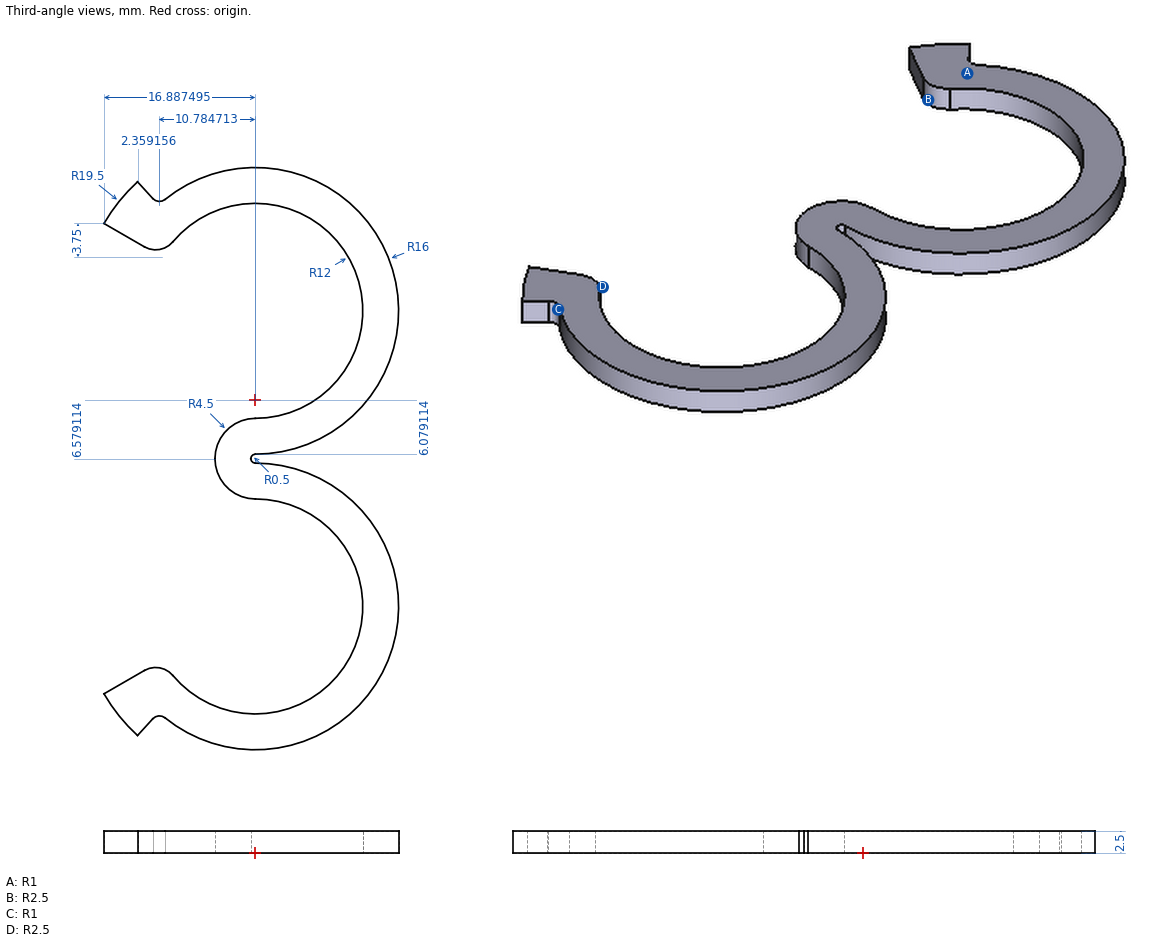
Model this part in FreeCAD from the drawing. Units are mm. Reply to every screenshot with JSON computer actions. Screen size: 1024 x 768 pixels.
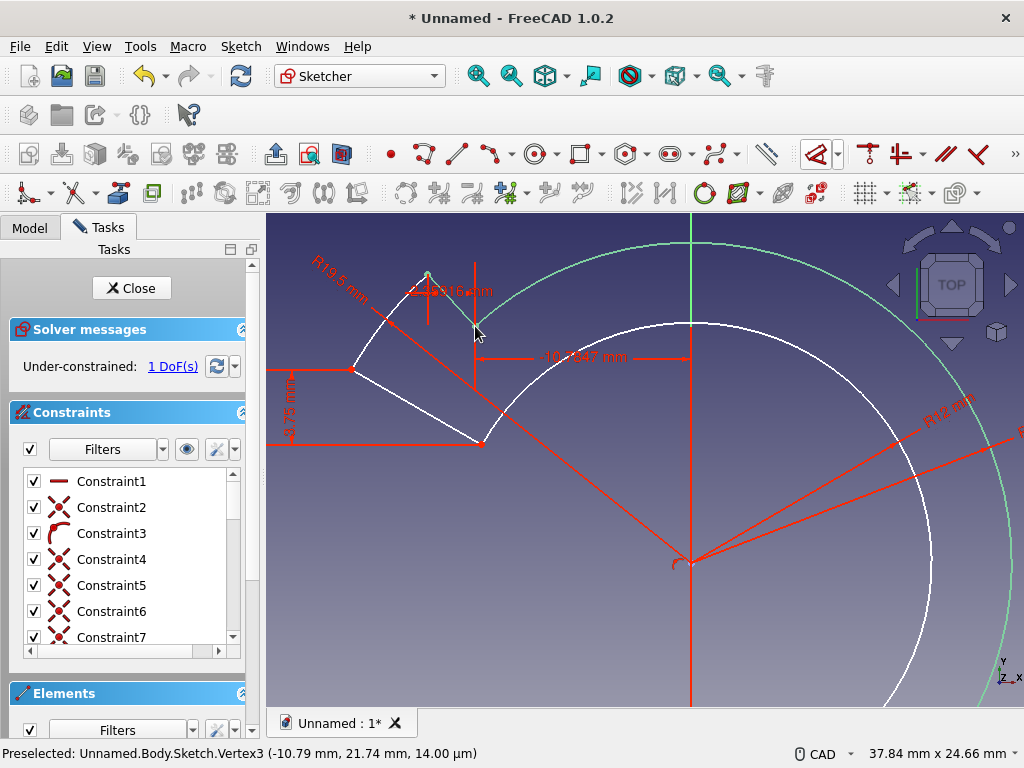
{"action": "left_click", "coordinate": [352, 370]}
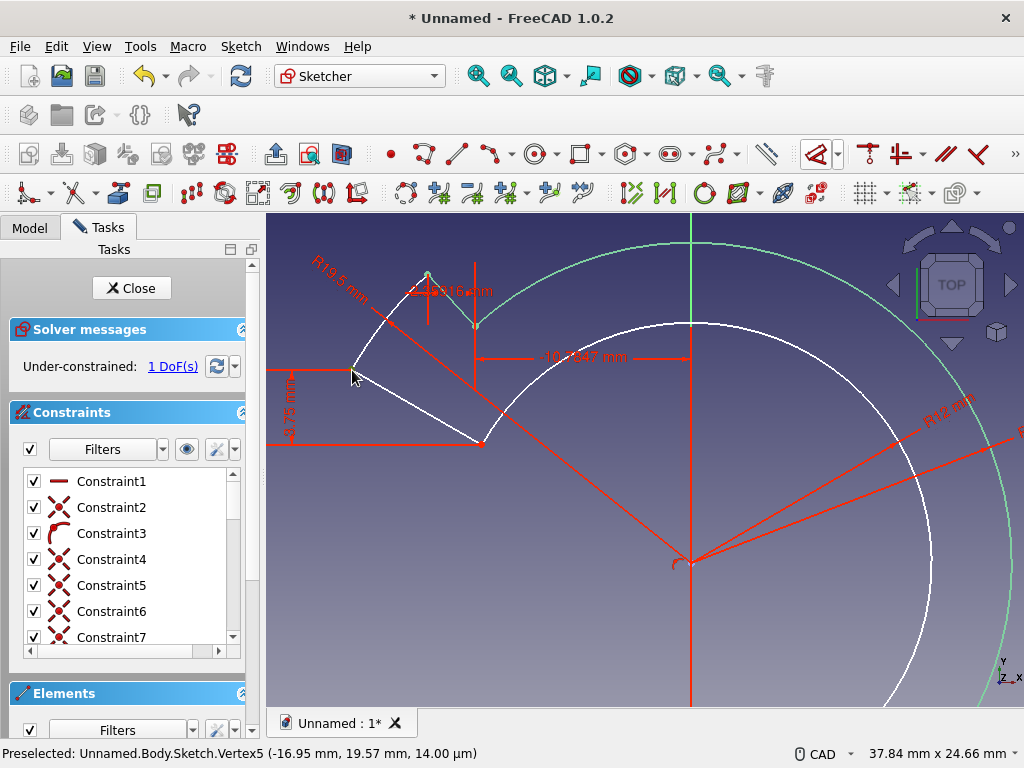
{"action": "left_click", "coordinate": [838, 154]}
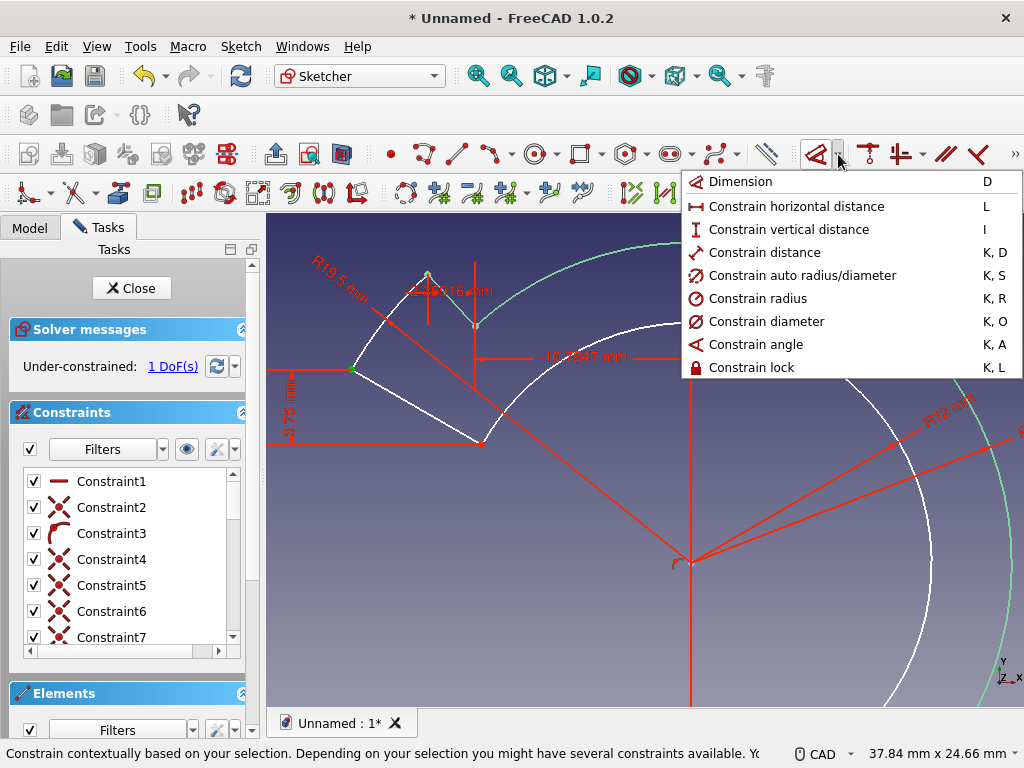
{"action": "left_click", "coordinate": [852, 206]}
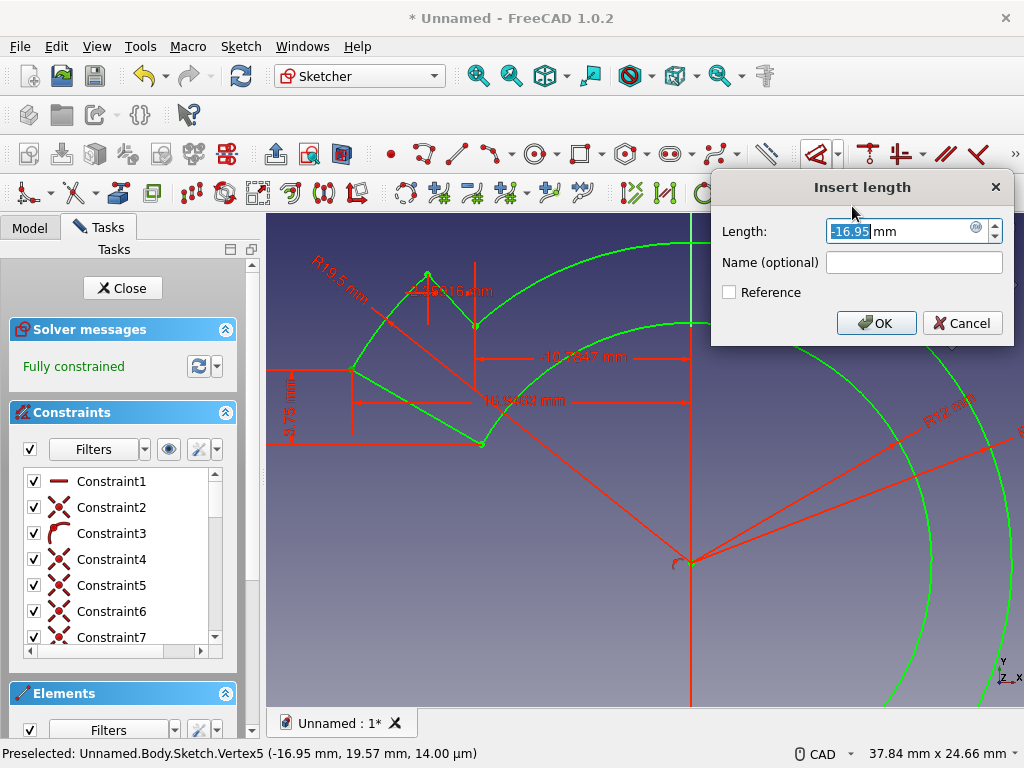
{"action": "type", "text": "-16.887495"}
{"action": "key", "text": "Return"}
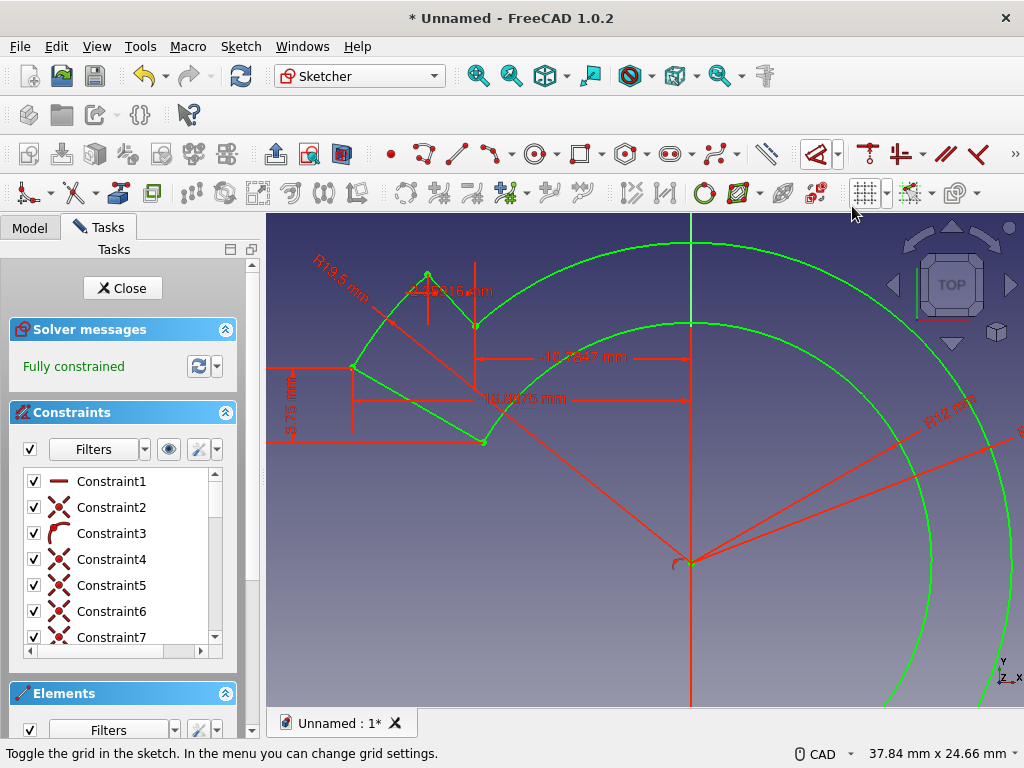
{"action": "left_click", "coordinate": [123, 288]}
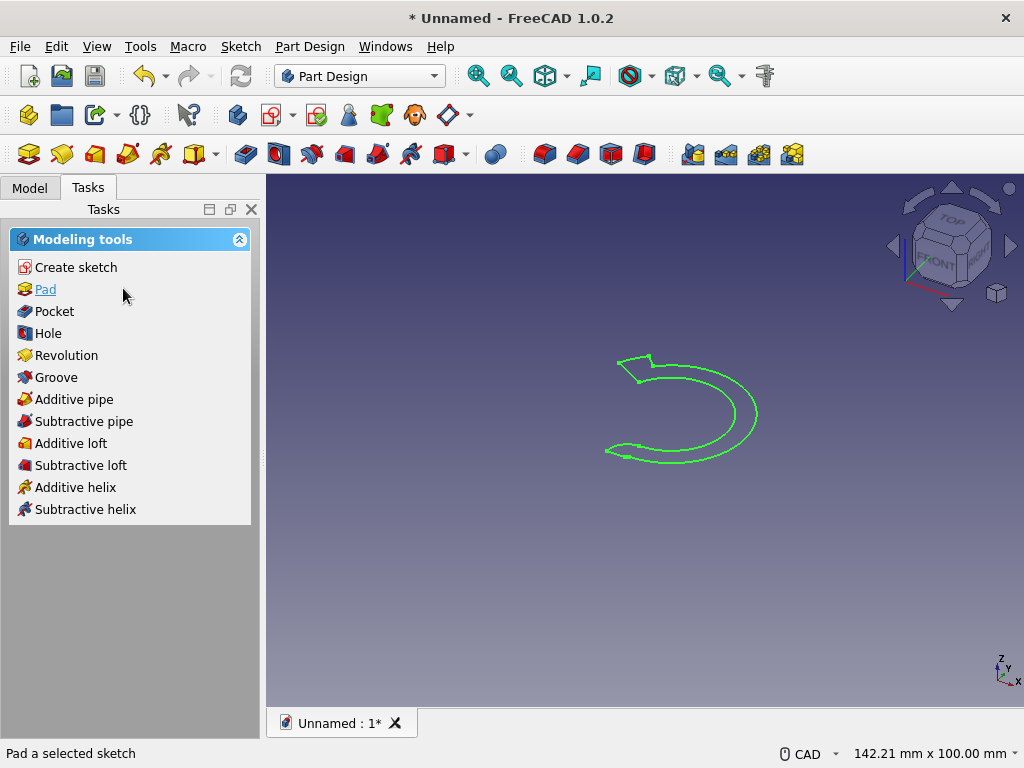
{"action": "left_click", "coordinate": [29, 154]}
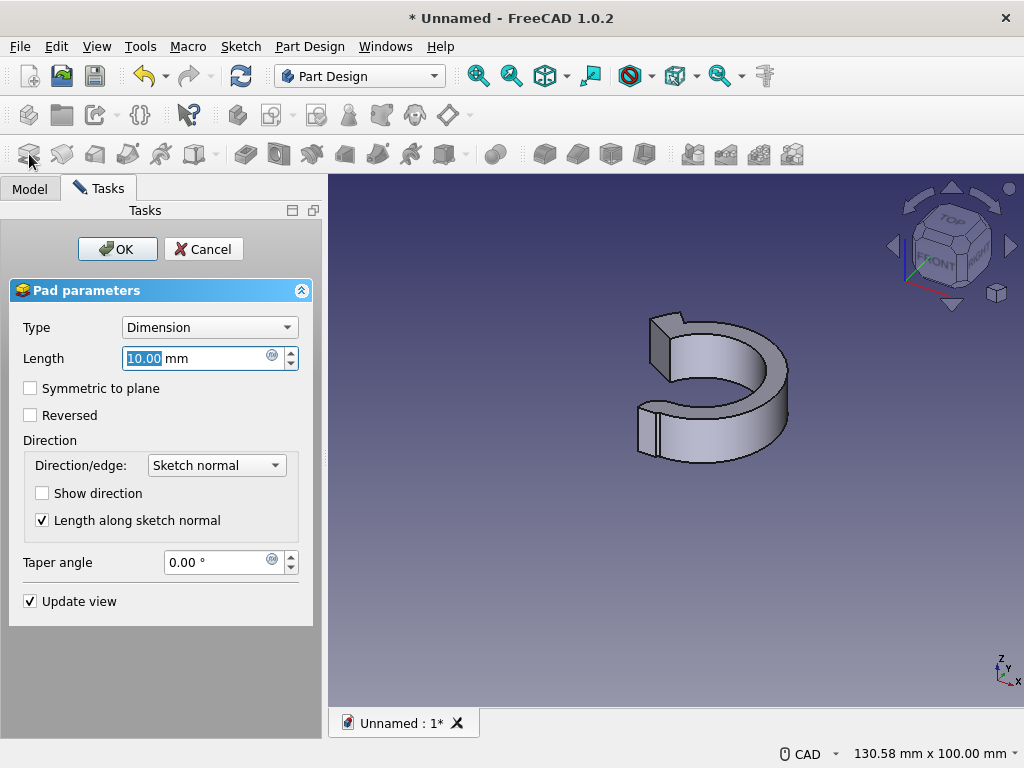
{"action": "type", "text": "2.5"}
{"action": "key", "text": "Tab"}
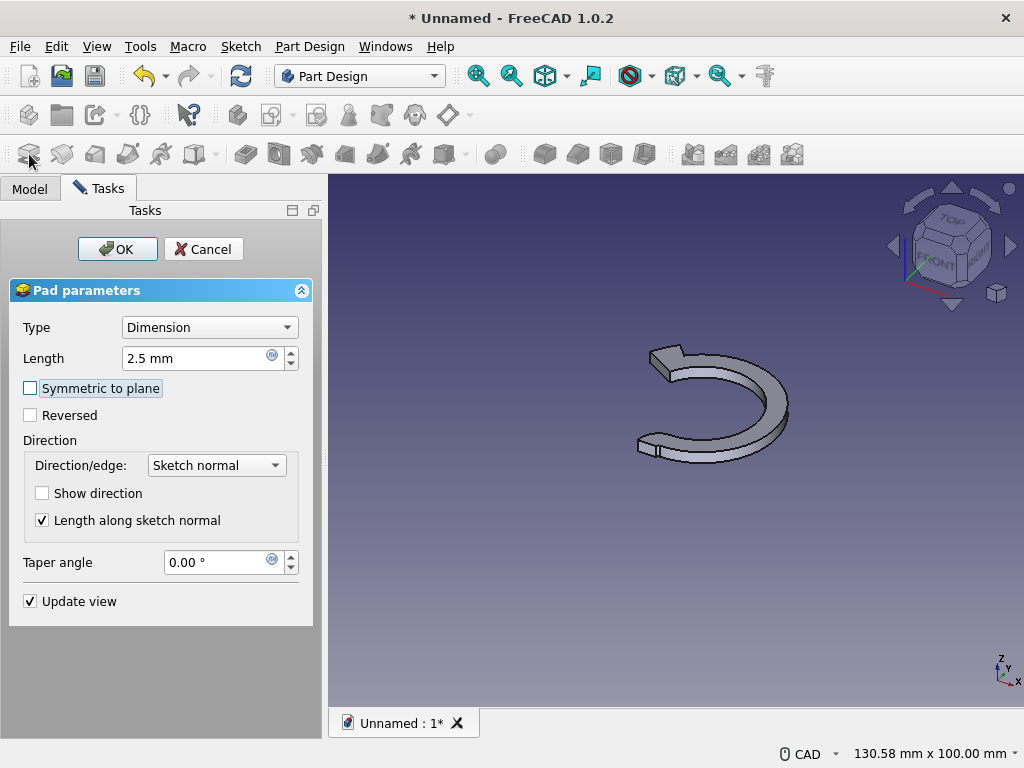
{"action": "left_click", "coordinate": [118, 249]}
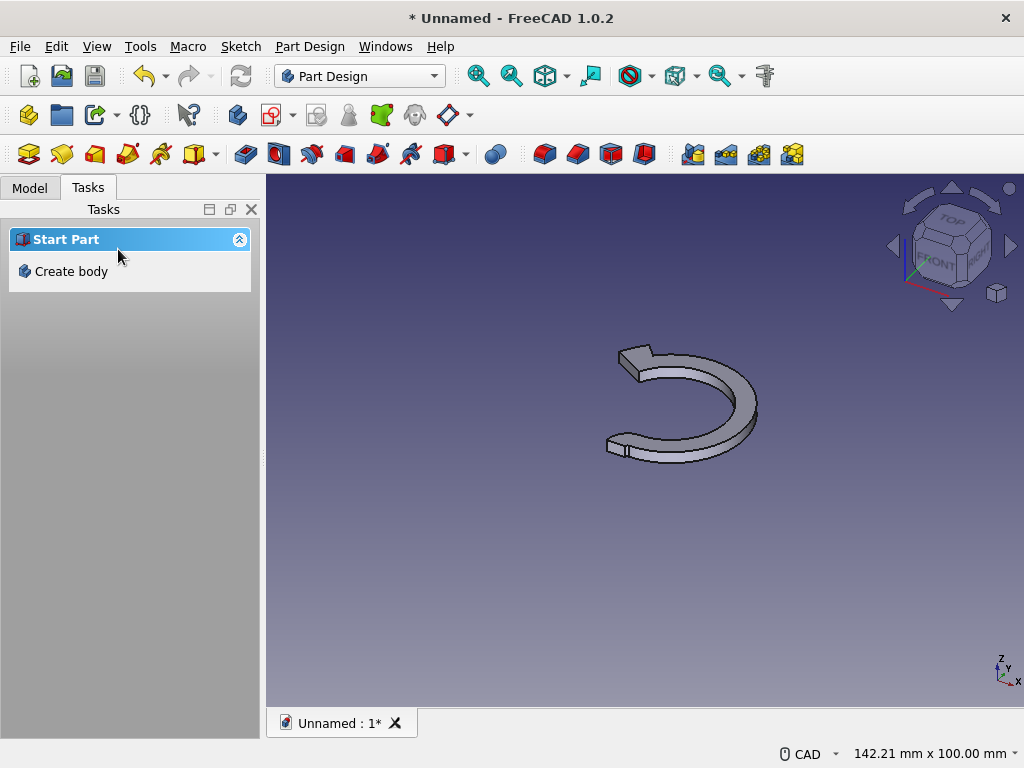
{"action": "left_click", "coordinate": [479, 76]}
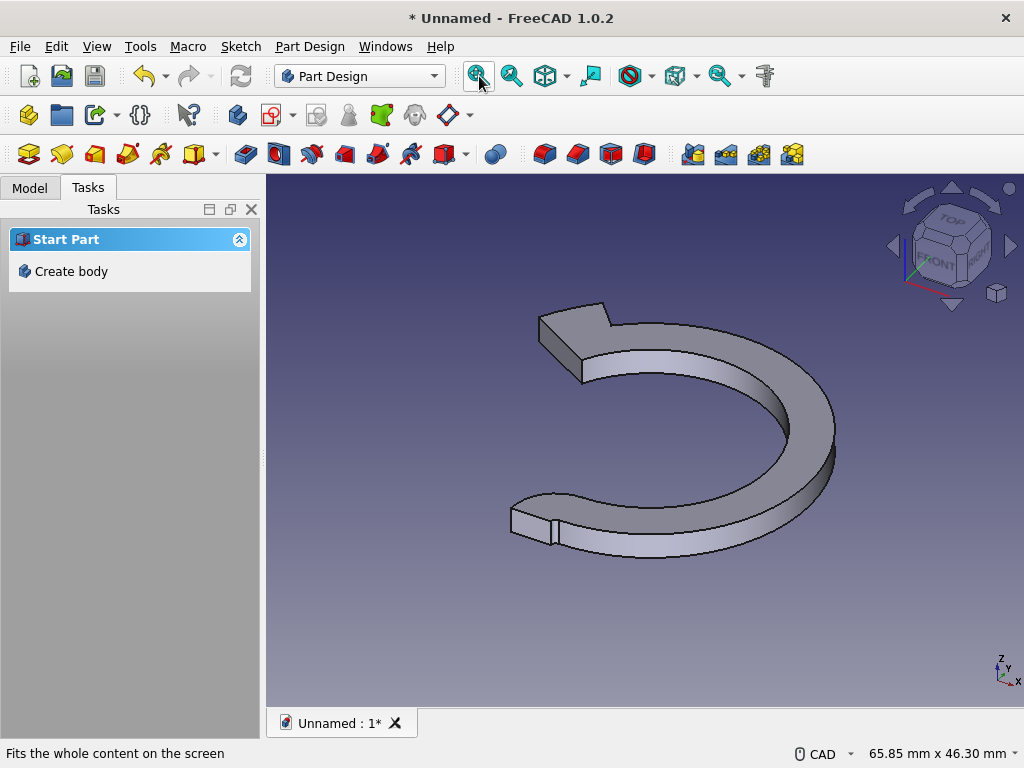
{"action": "key", "text": "0"}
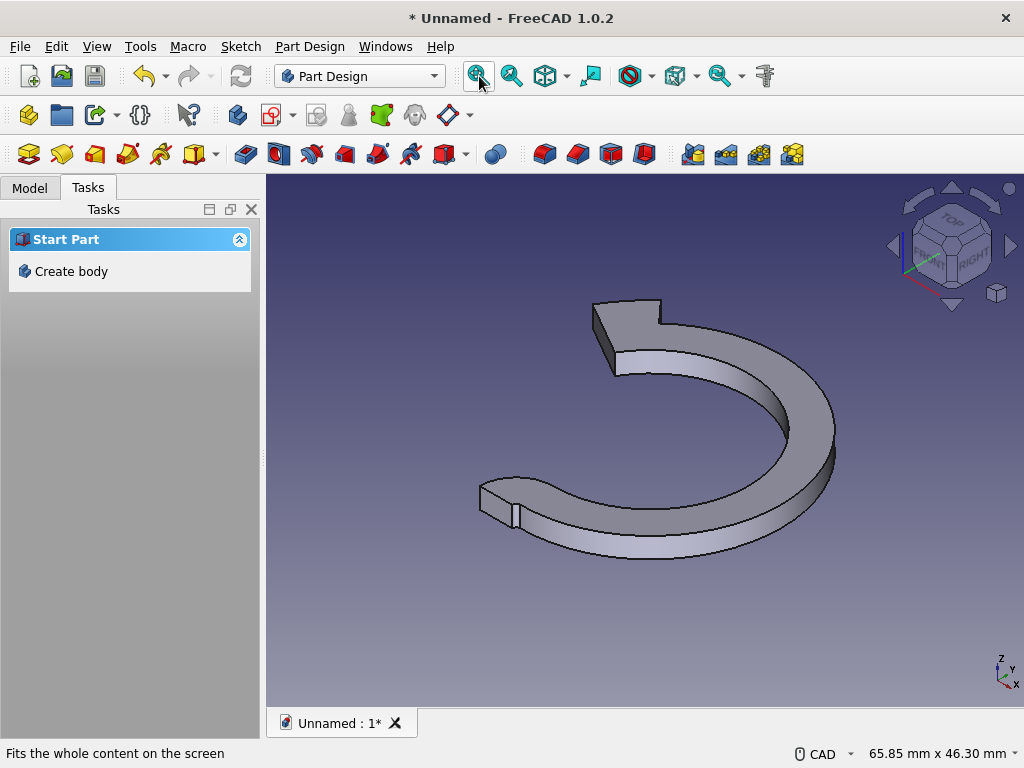
{"action": "key", "text": "2"}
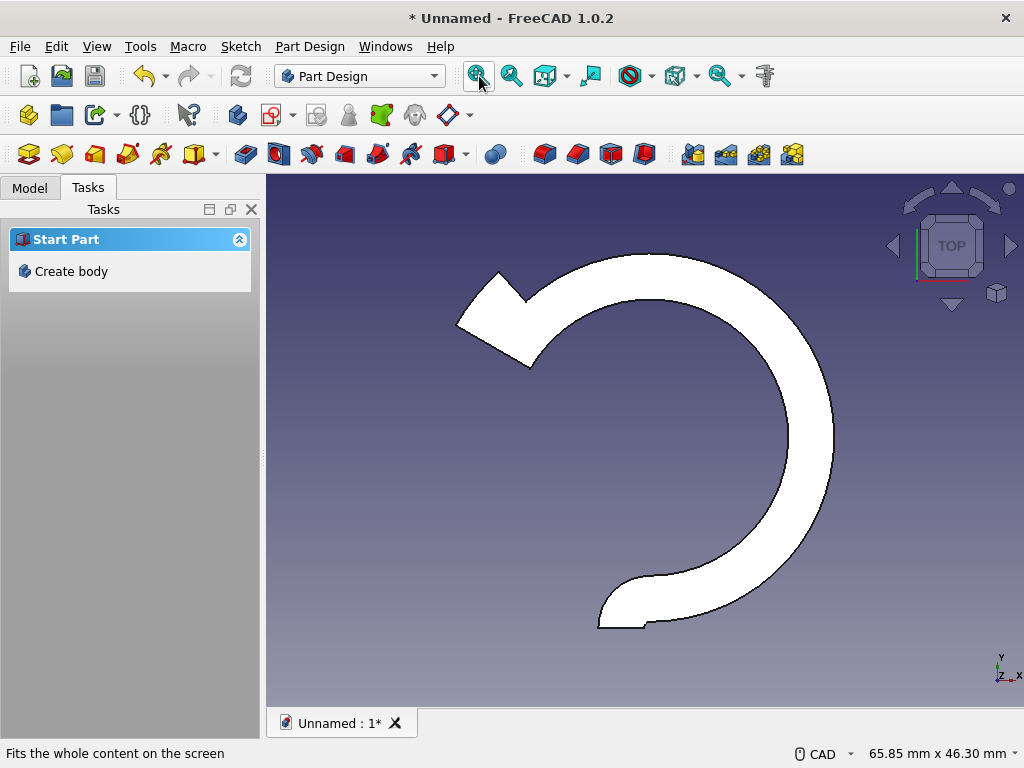
{"action": "key", "text": "1"}